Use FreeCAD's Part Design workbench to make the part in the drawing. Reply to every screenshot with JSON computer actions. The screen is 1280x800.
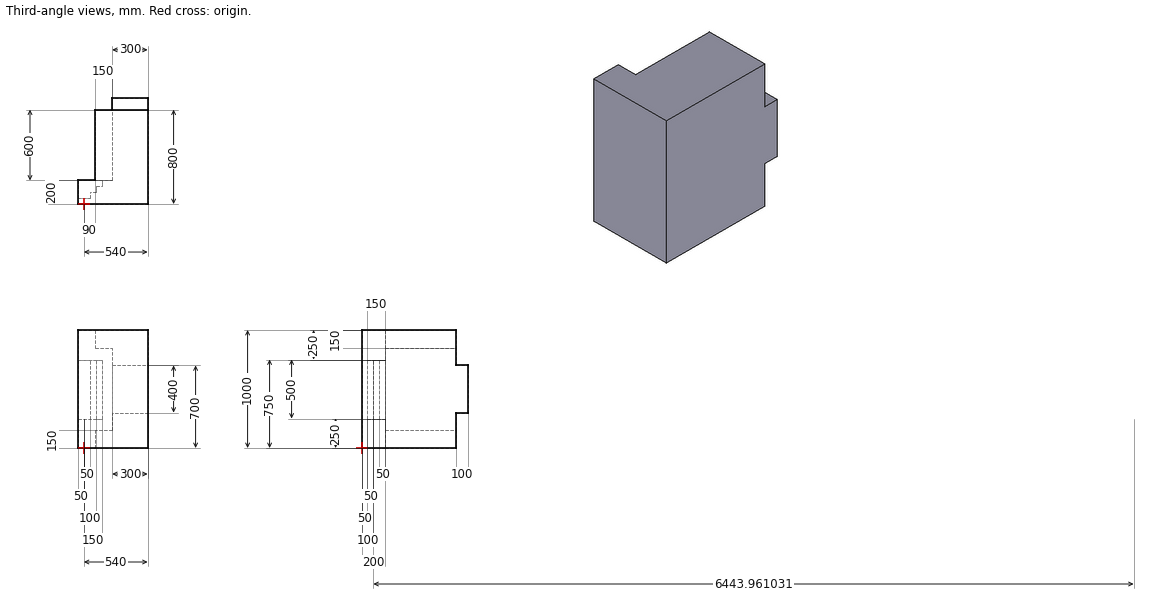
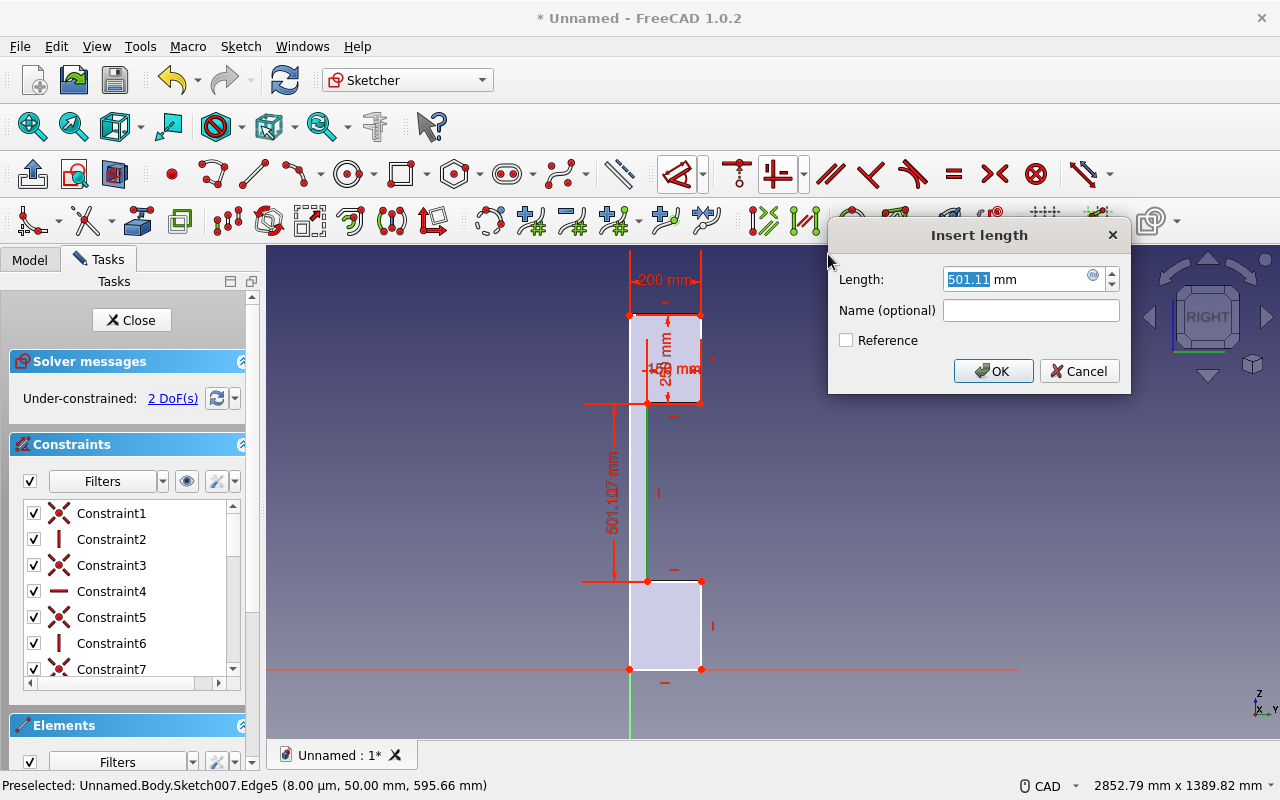
{"action": "type", "text": "500"}
{"action": "key", "text": "Return"}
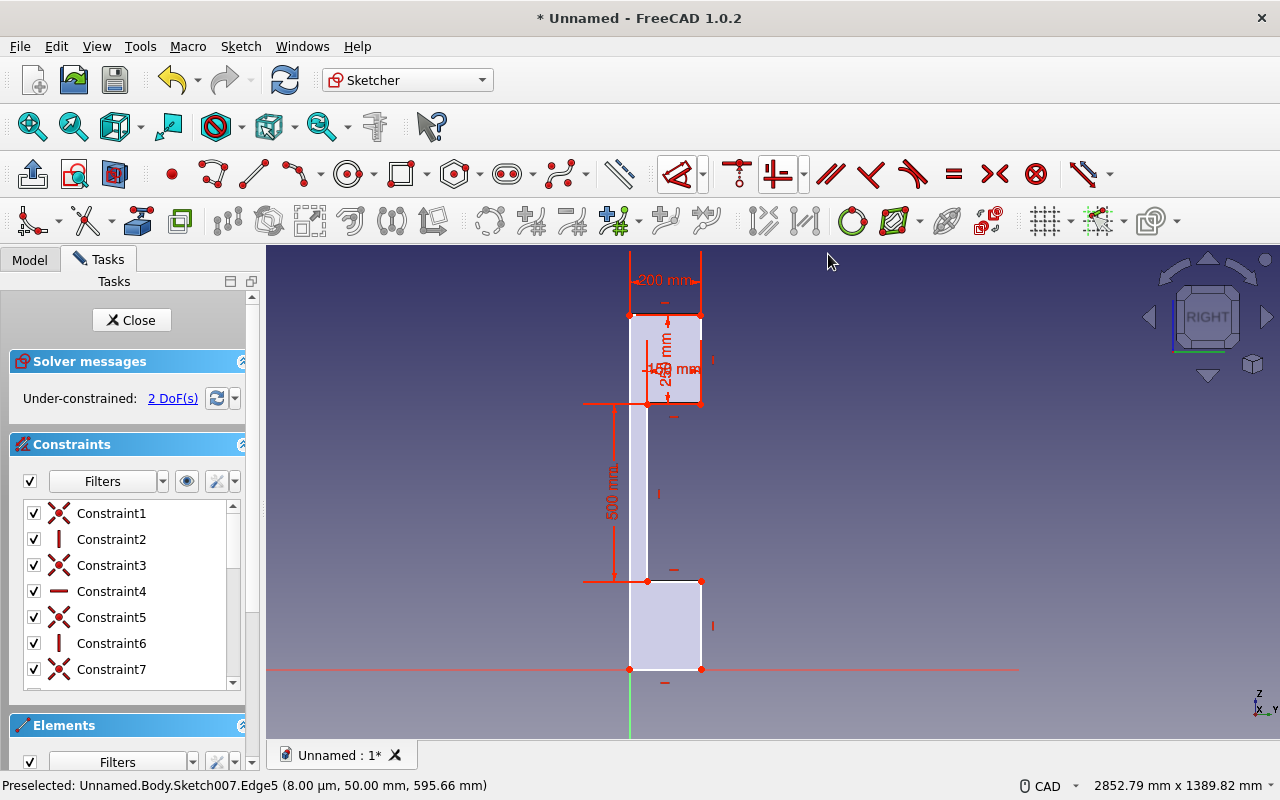
{"action": "left_click", "coordinate": [663, 582]}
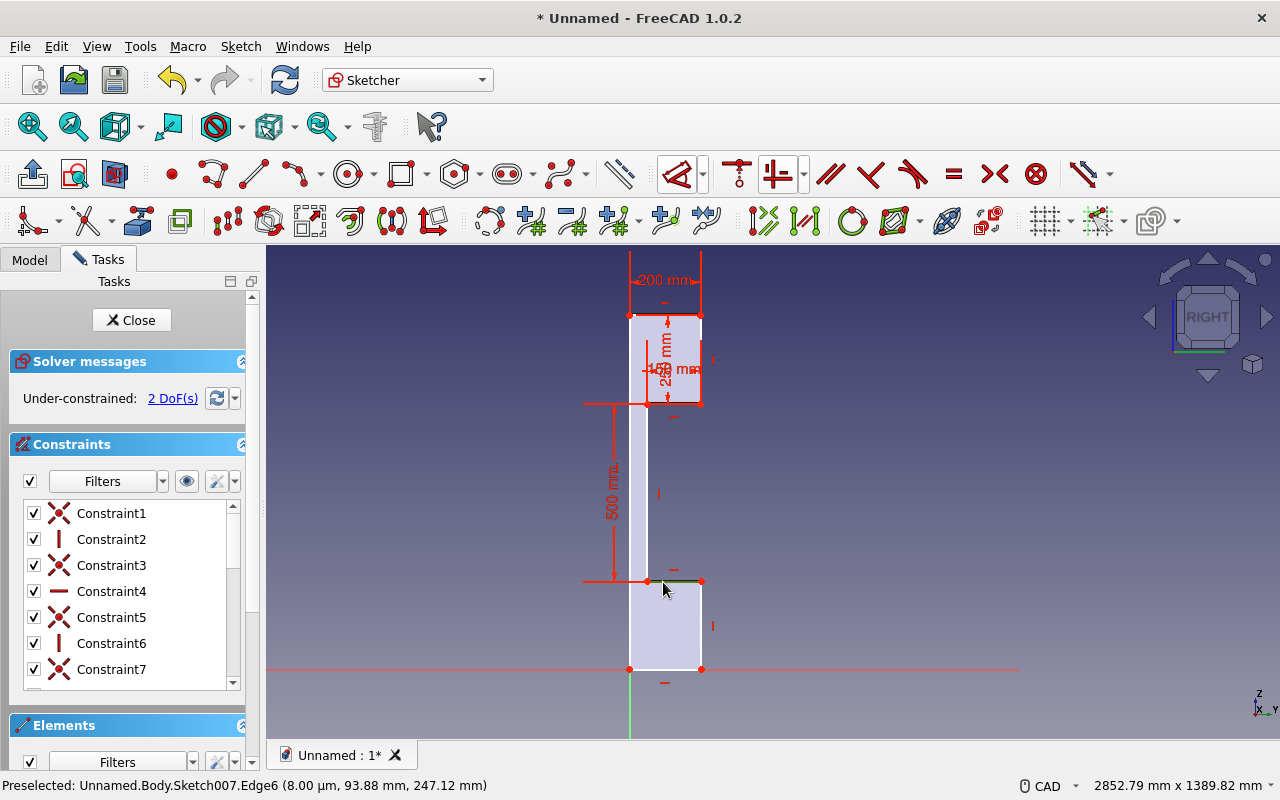
{"action": "left_click", "coordinate": [702, 174]}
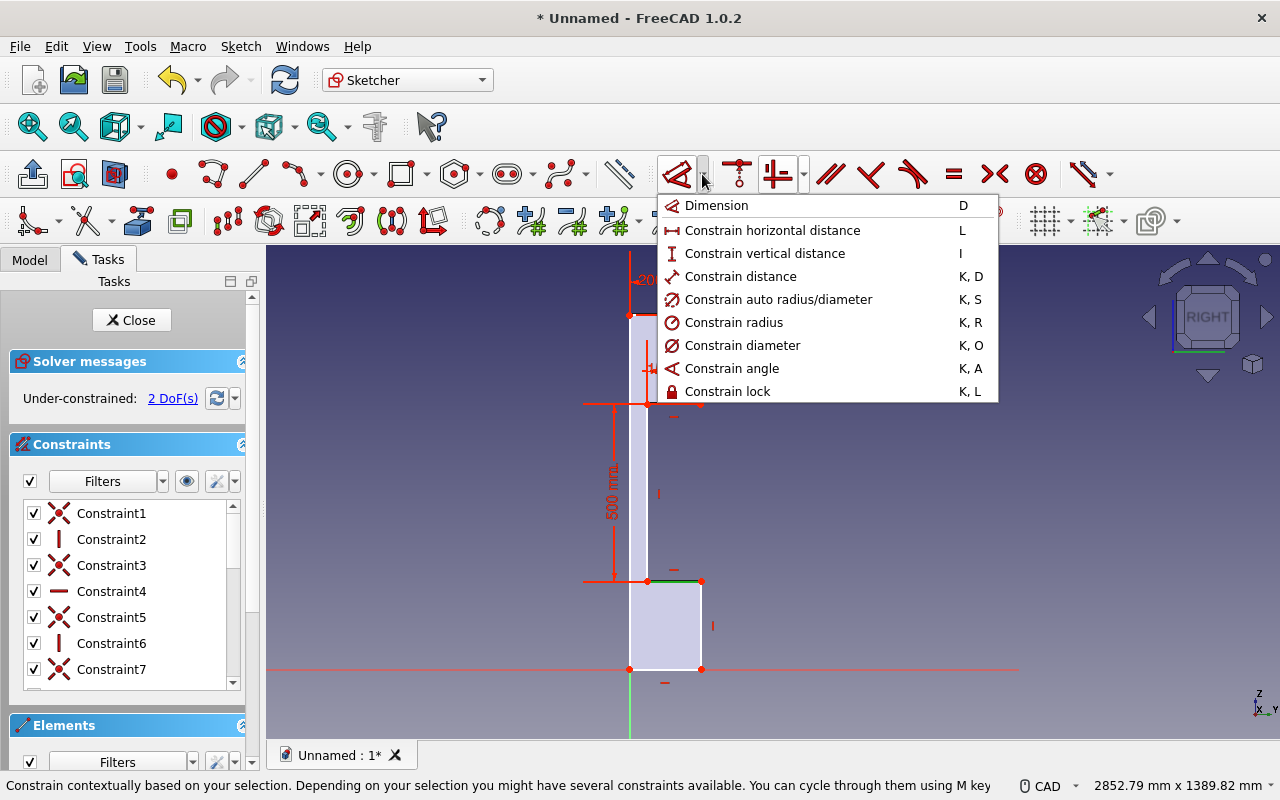
{"action": "left_click", "coordinate": [828, 230]}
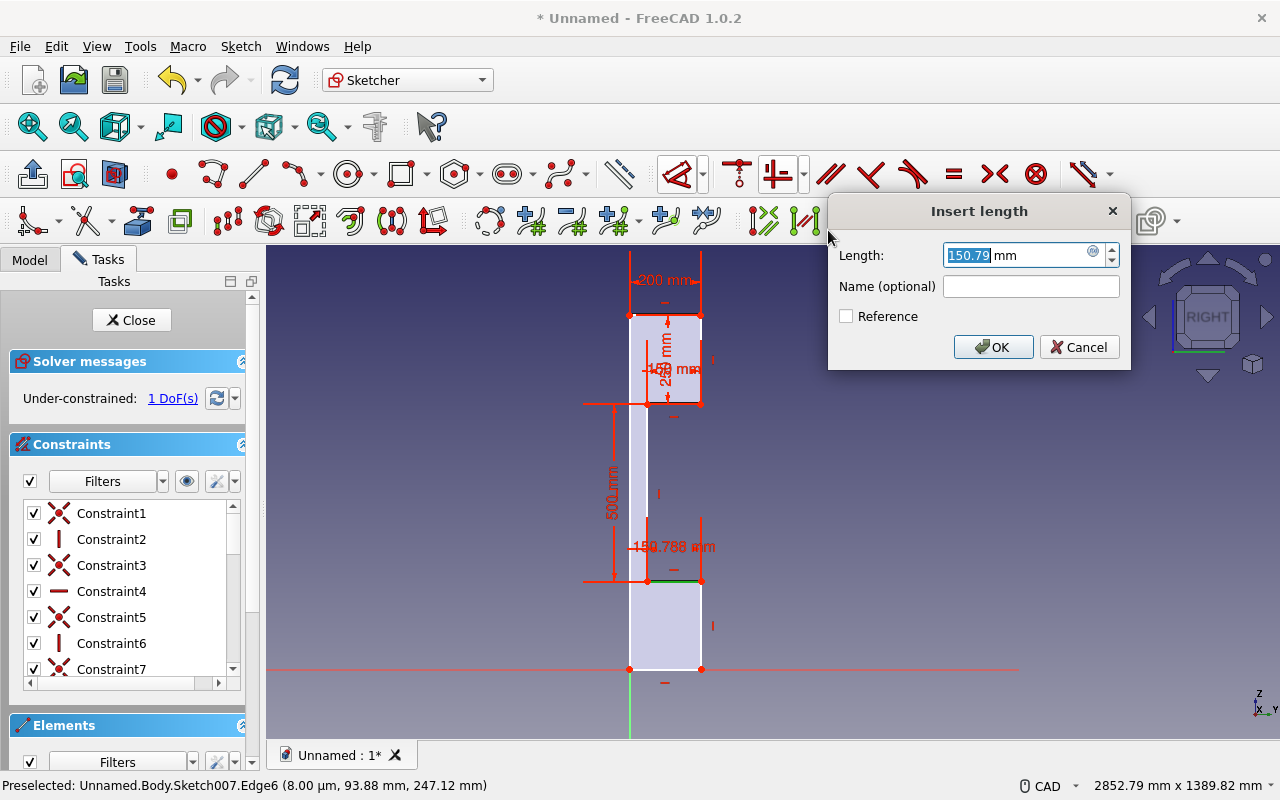
{"action": "type", "text": "150"}
{"action": "key", "text": "Return"}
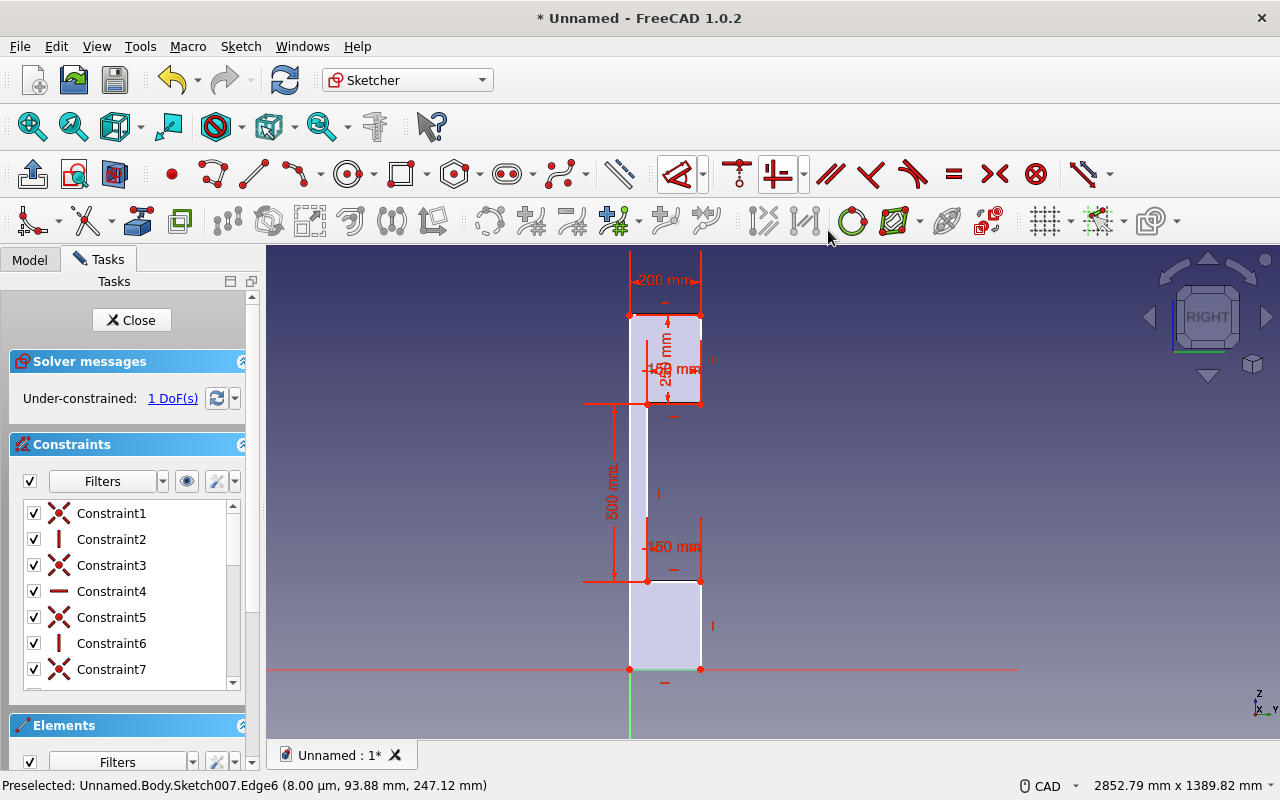
{"action": "left_click", "coordinate": [701, 608]}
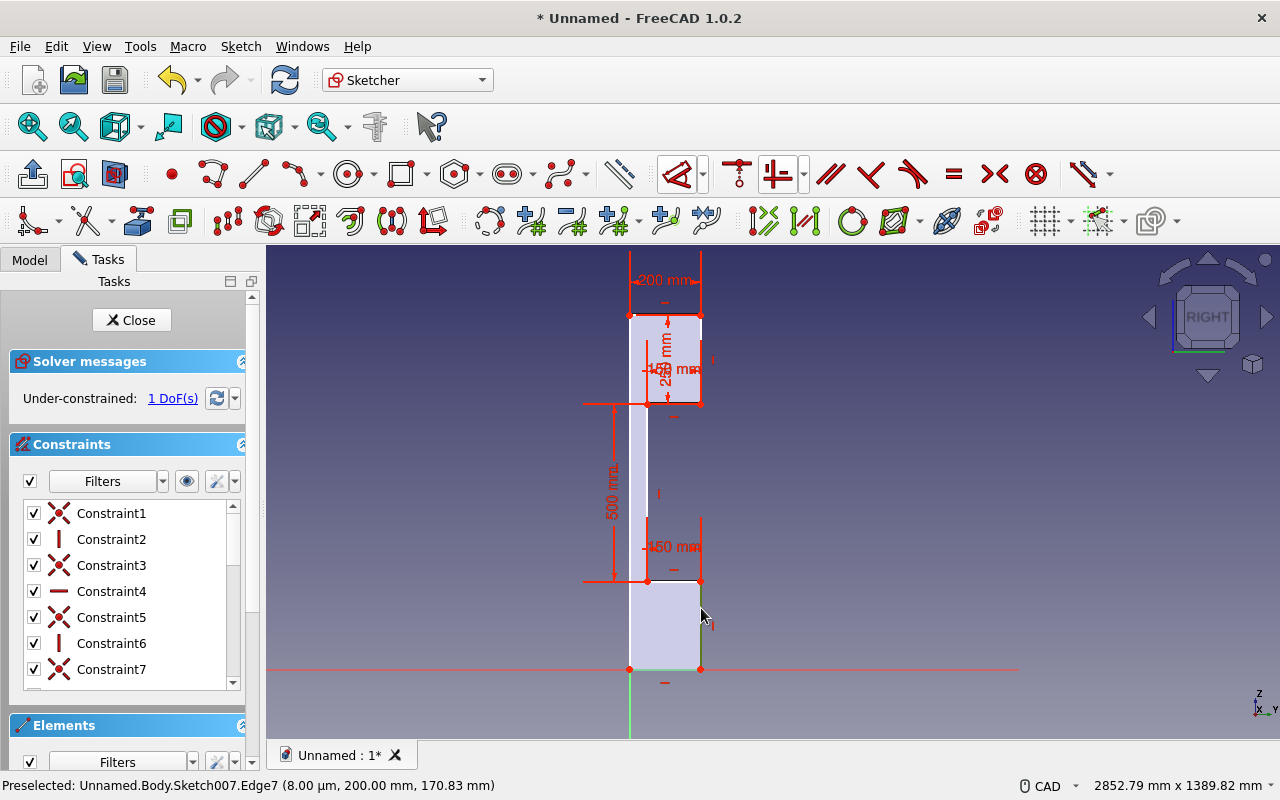
{"action": "left_click", "coordinate": [702, 174]}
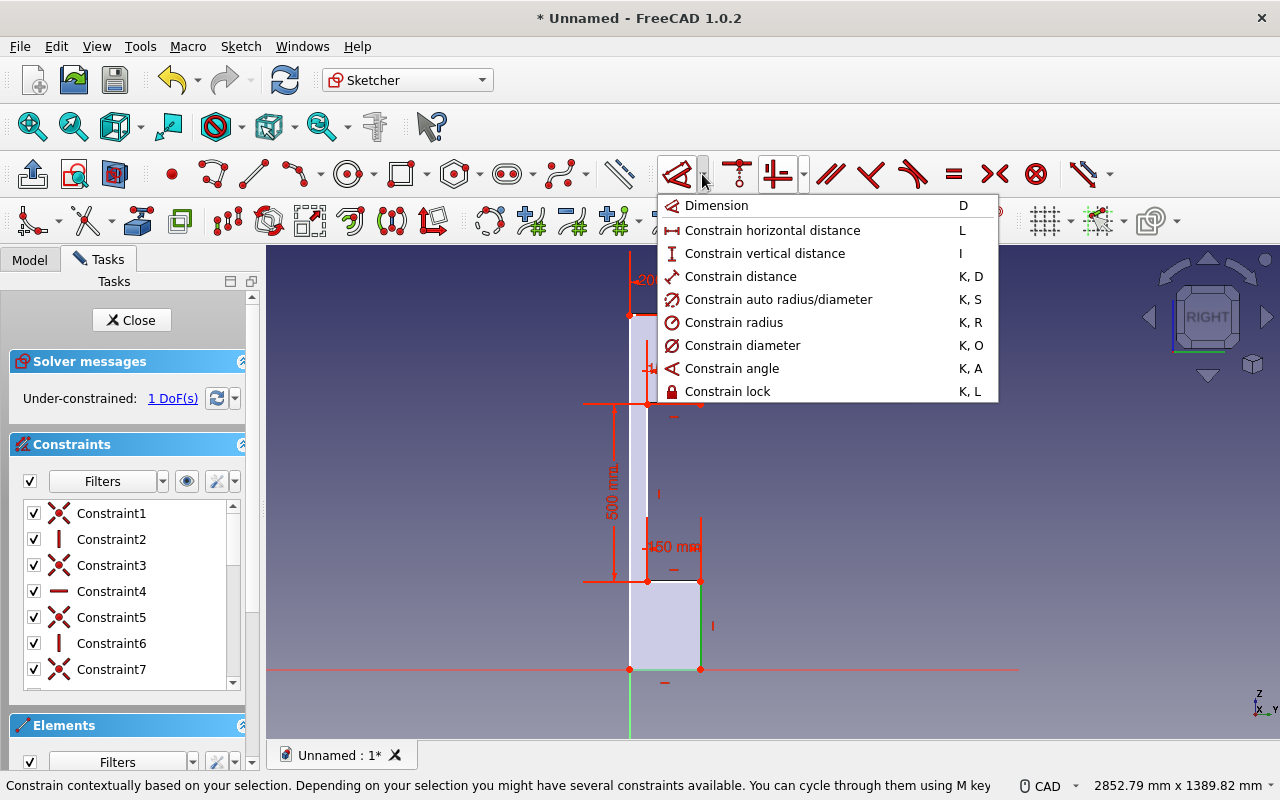
{"action": "left_click", "coordinate": [828, 254]}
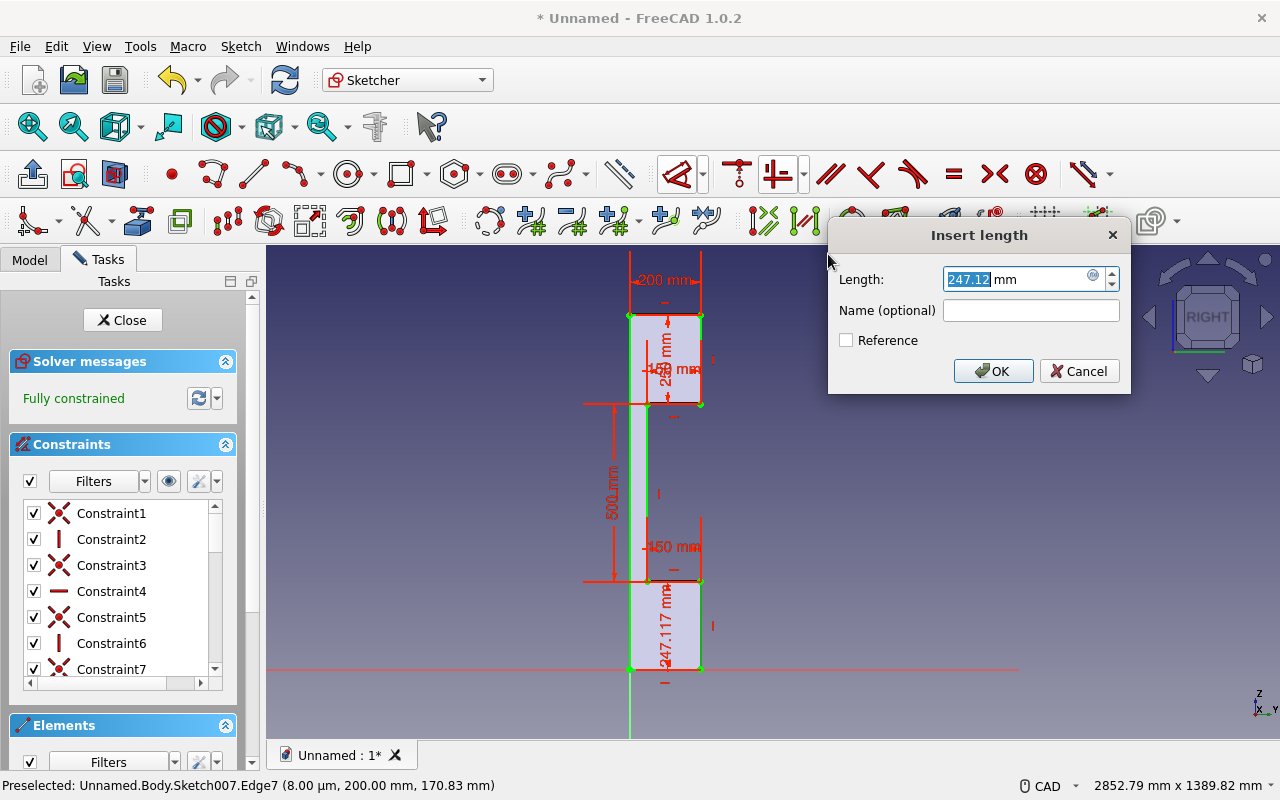
{"action": "type", "text": "250"}
{"action": "key", "text": "Return"}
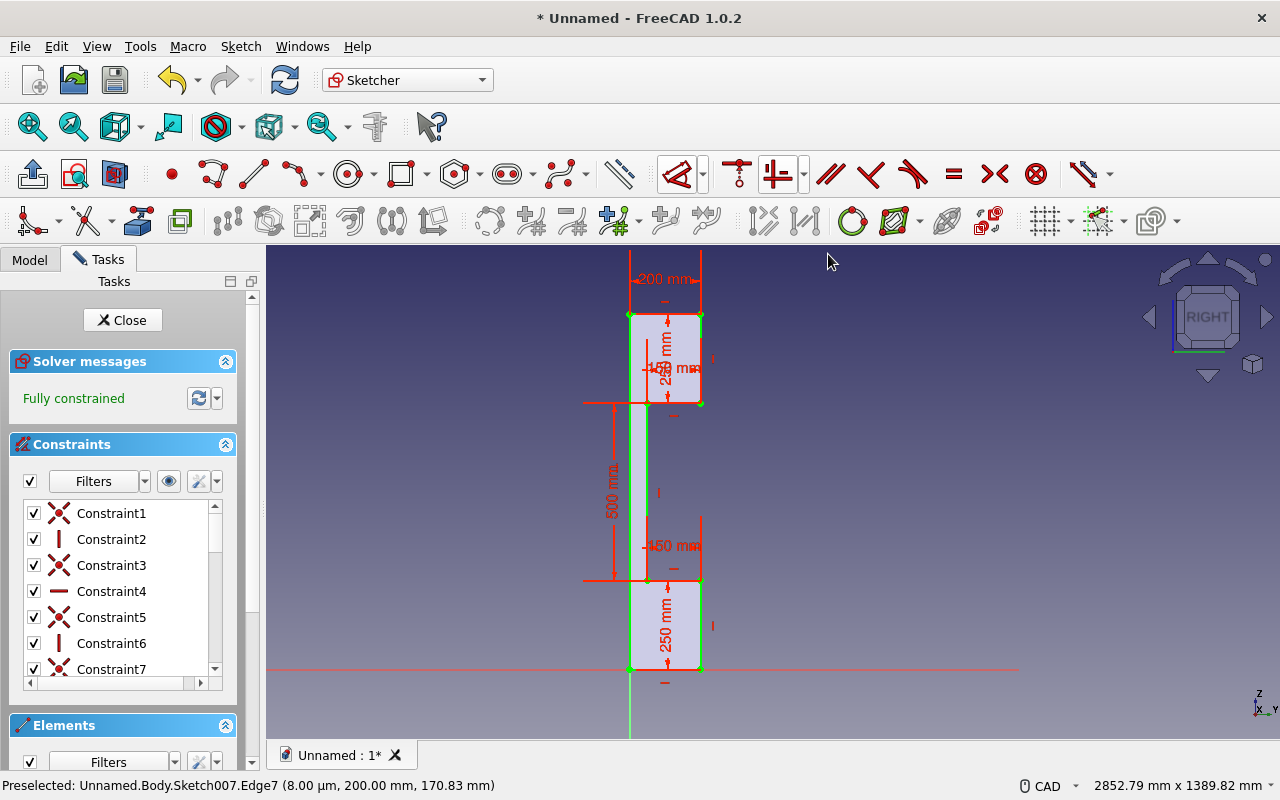
{"action": "left_click", "coordinate": [123, 320]}